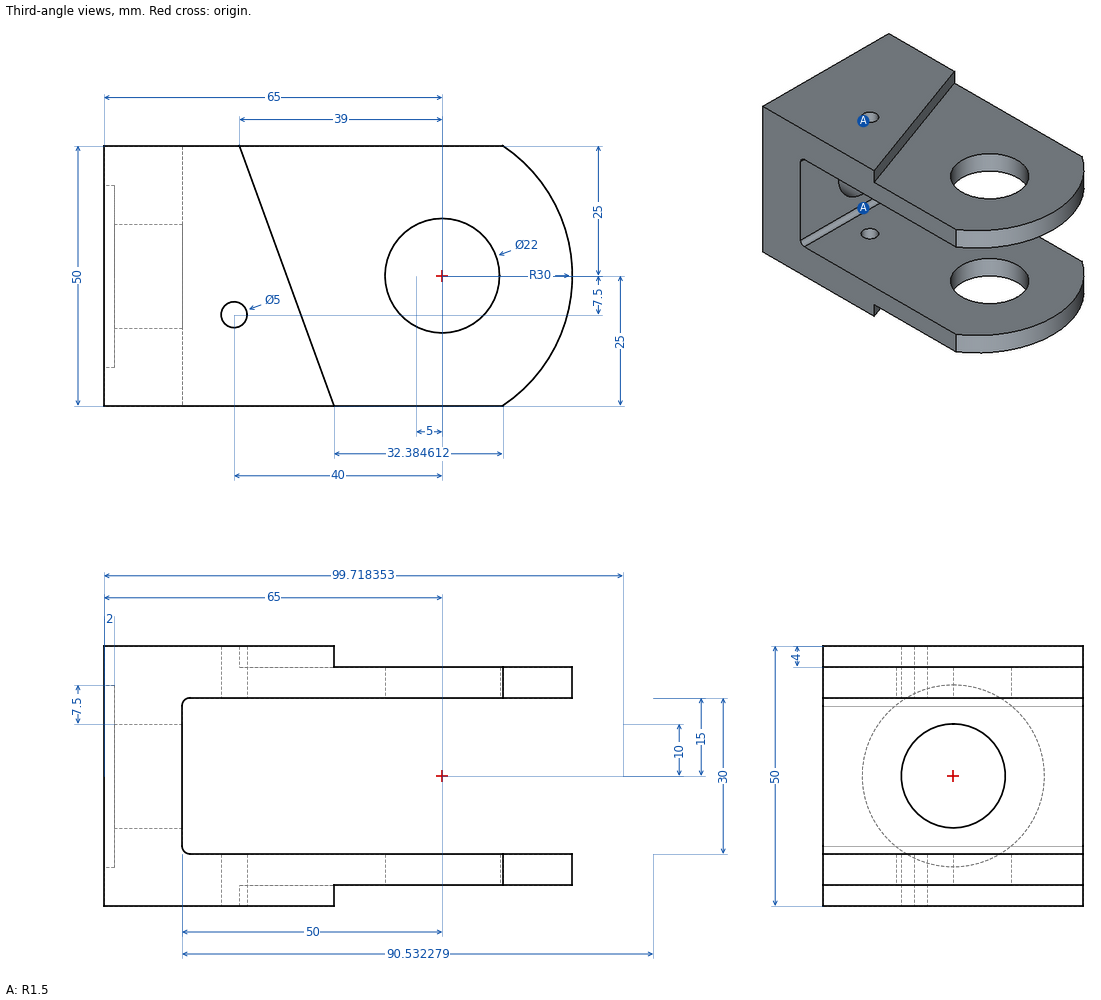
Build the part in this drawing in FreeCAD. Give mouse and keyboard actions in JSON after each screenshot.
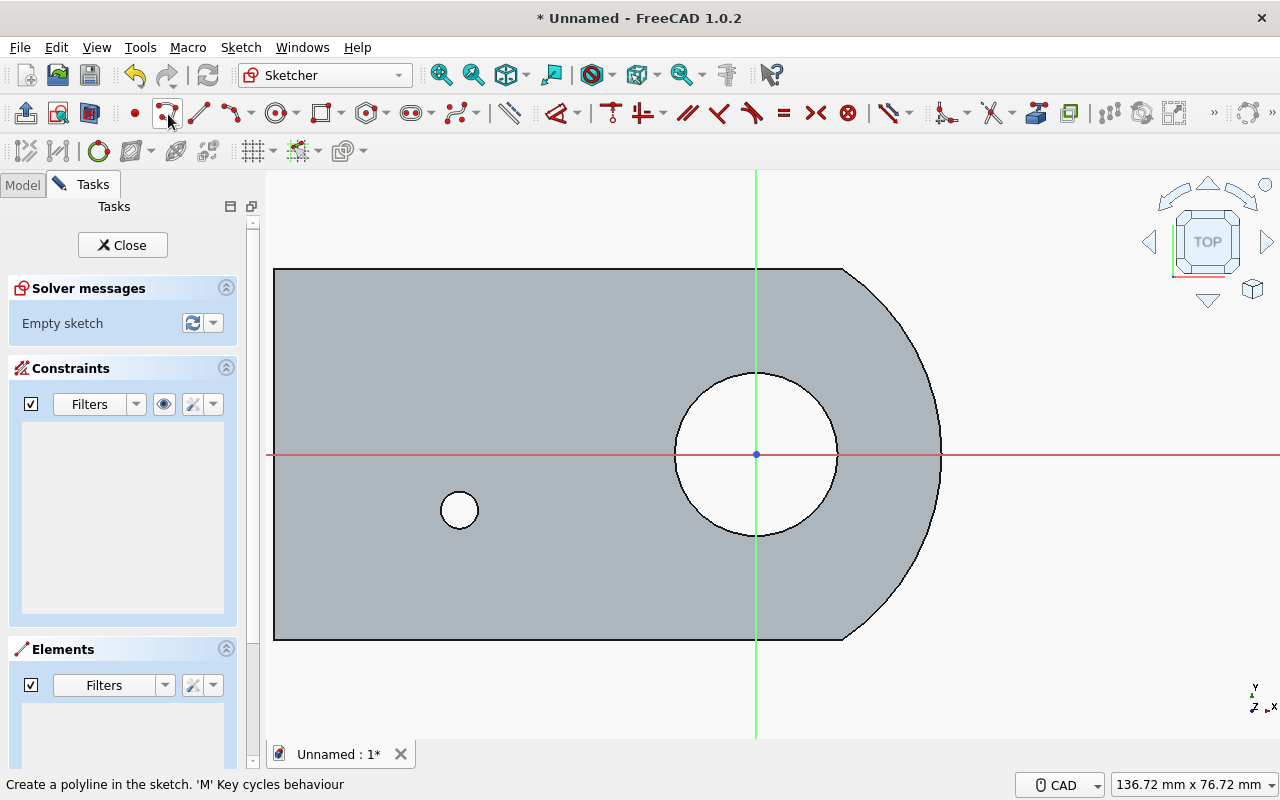
{"action": "left_click", "coordinate": [842, 269]}
{"action": "left_click", "coordinate": [467, 269]}
{"action": "left_click", "coordinate": [602, 640]}
{"action": "left_click", "coordinate": [842, 640]}
{"action": "right_click", "coordinate": [842, 640]}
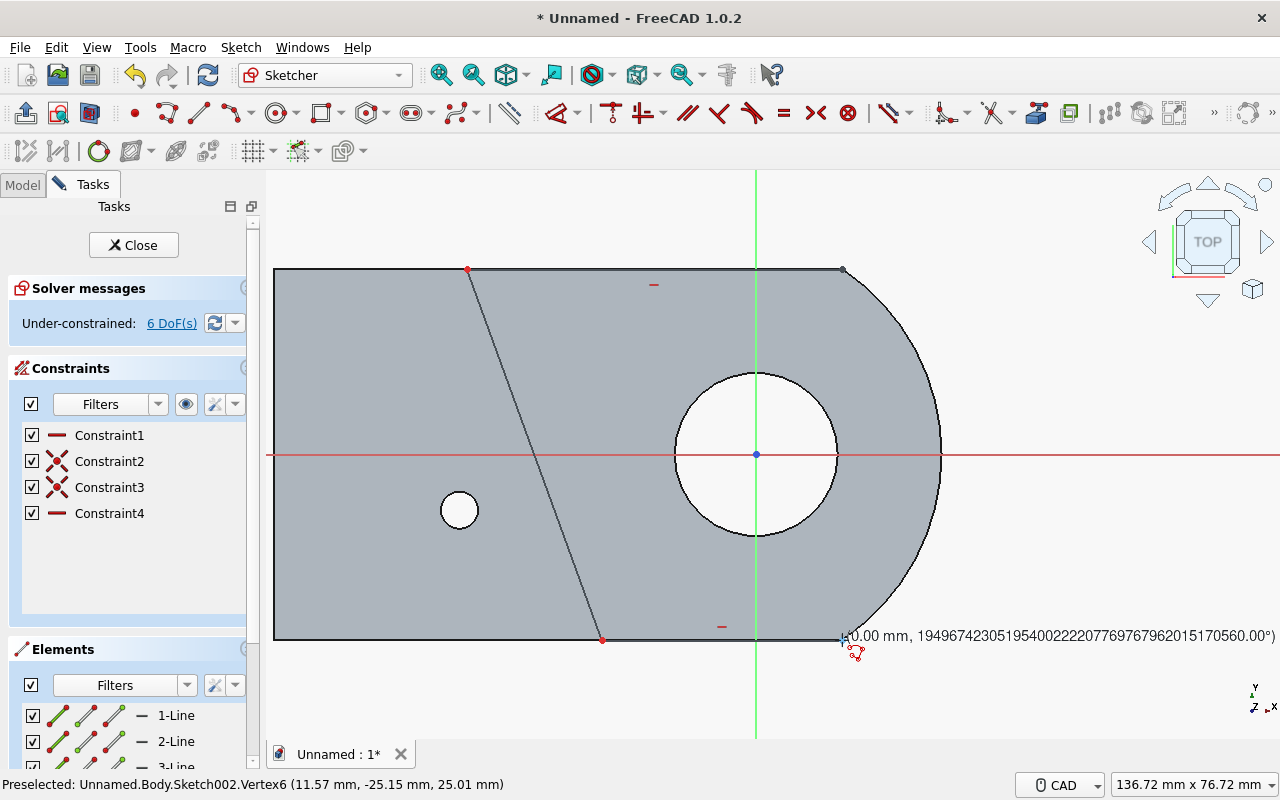
{"action": "left_click", "coordinate": [232, 114]}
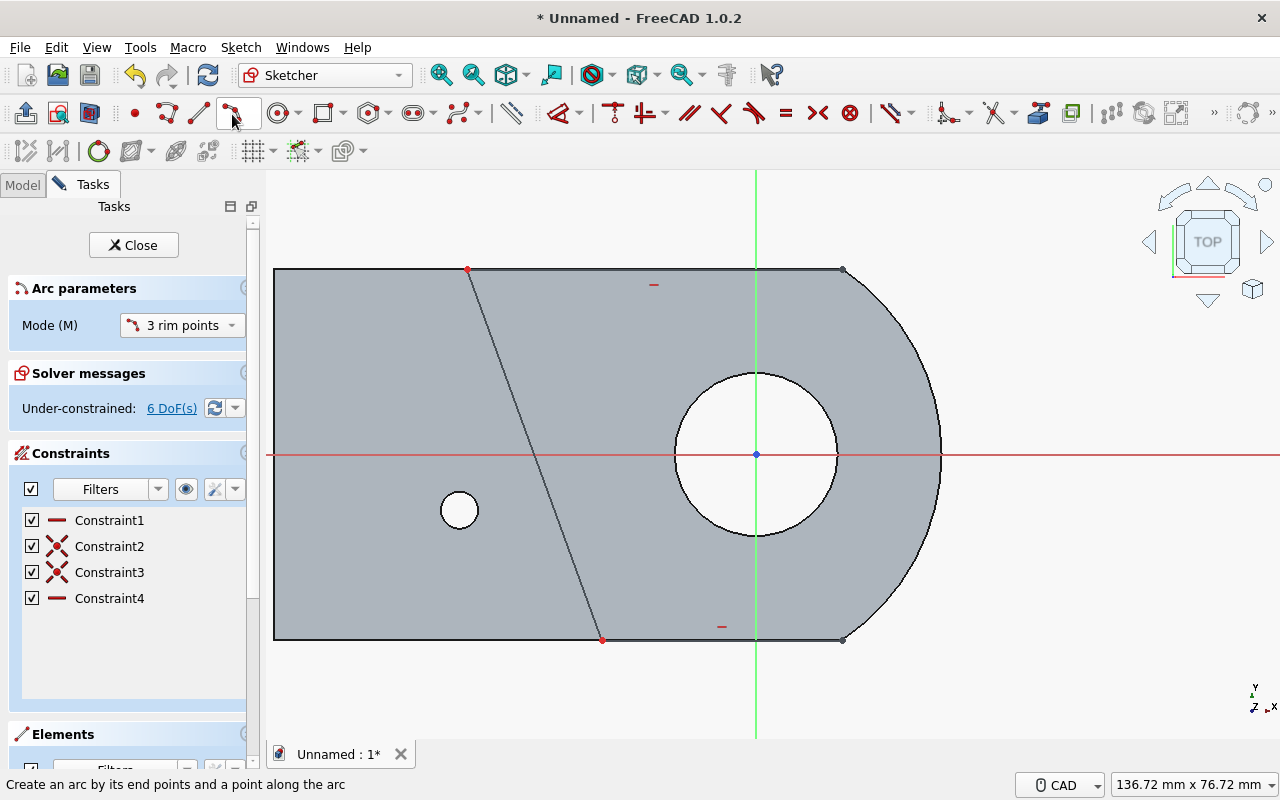
{"action": "left_click", "coordinate": [842, 641]}
{"action": "left_click", "coordinate": [842, 270]}
{"action": "left_click", "coordinate": [937, 498]}
{"action": "key", "text": "Escape"}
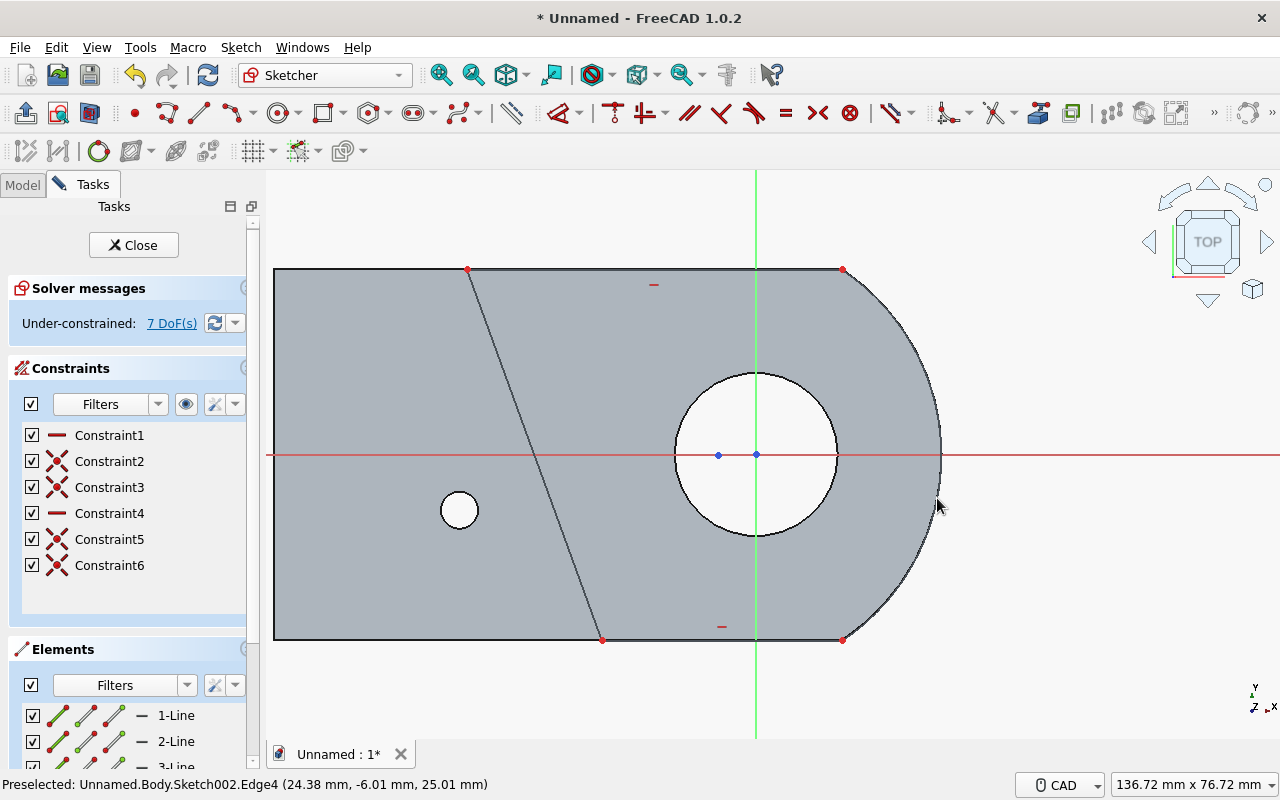
{"action": "left_click", "coordinate": [718, 455]}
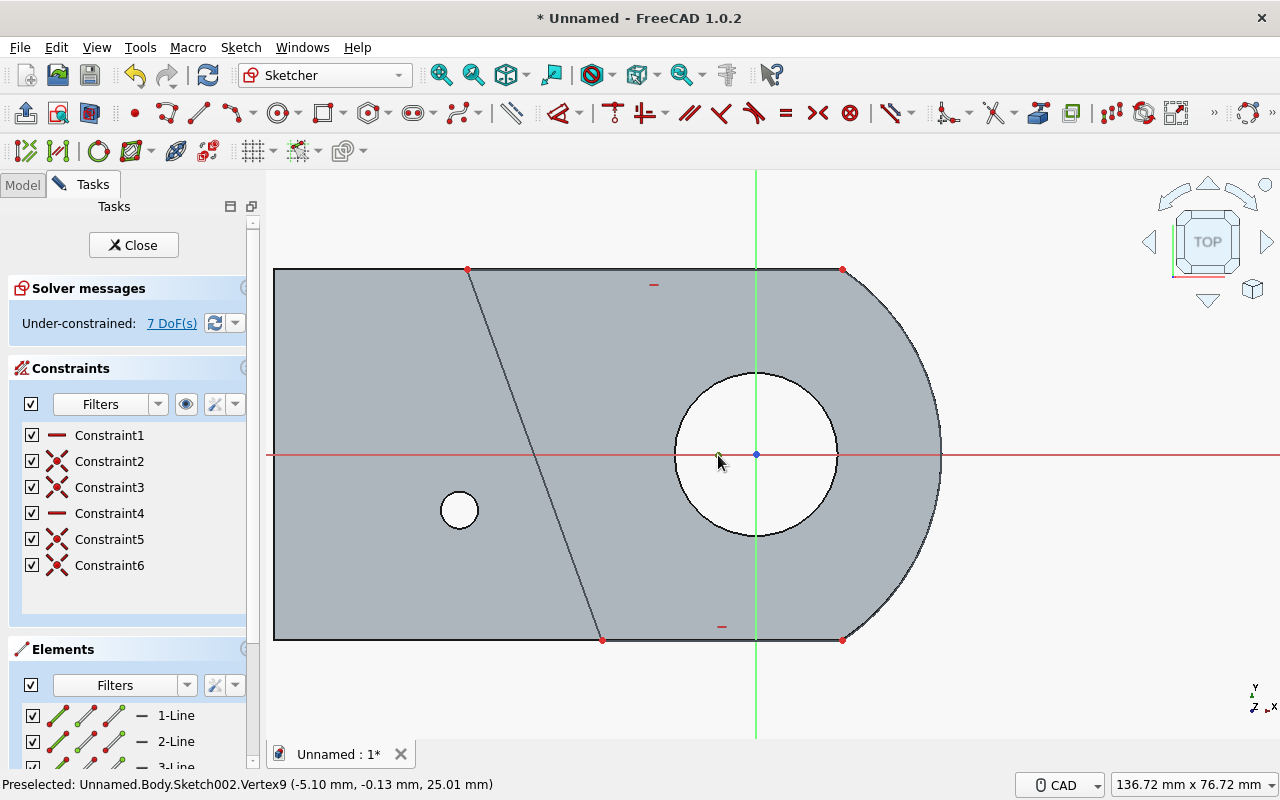
{"action": "left_click", "coordinate": [353, 454]}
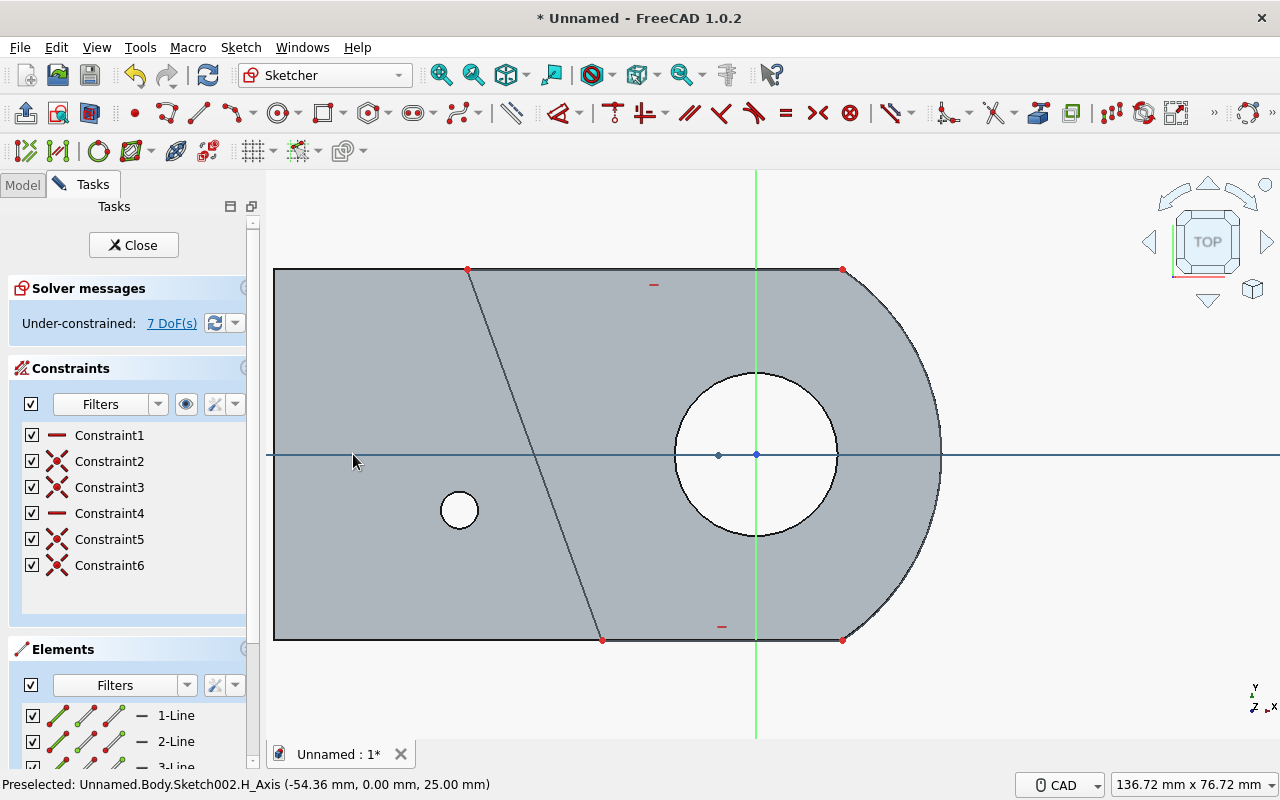
{"action": "left_click", "coordinate": [614, 114]}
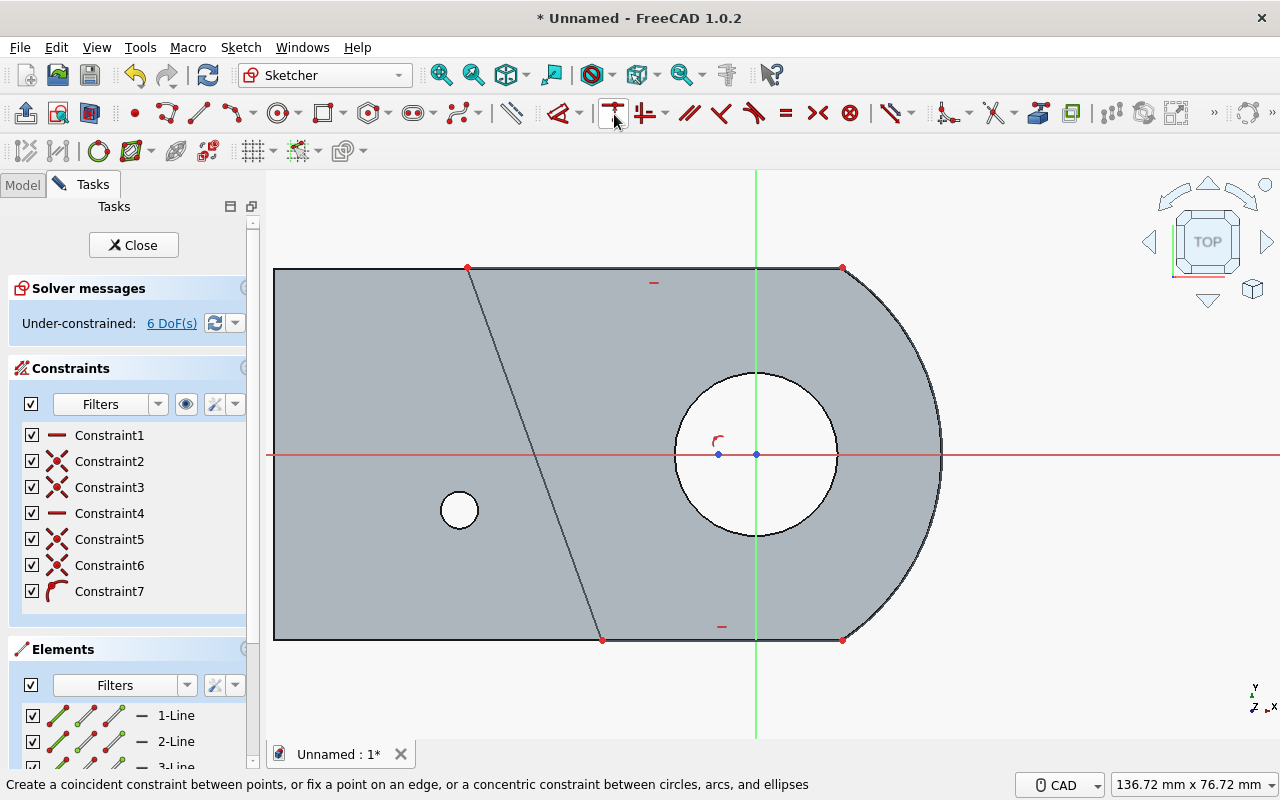
{"action": "left_click", "coordinate": [558, 114]}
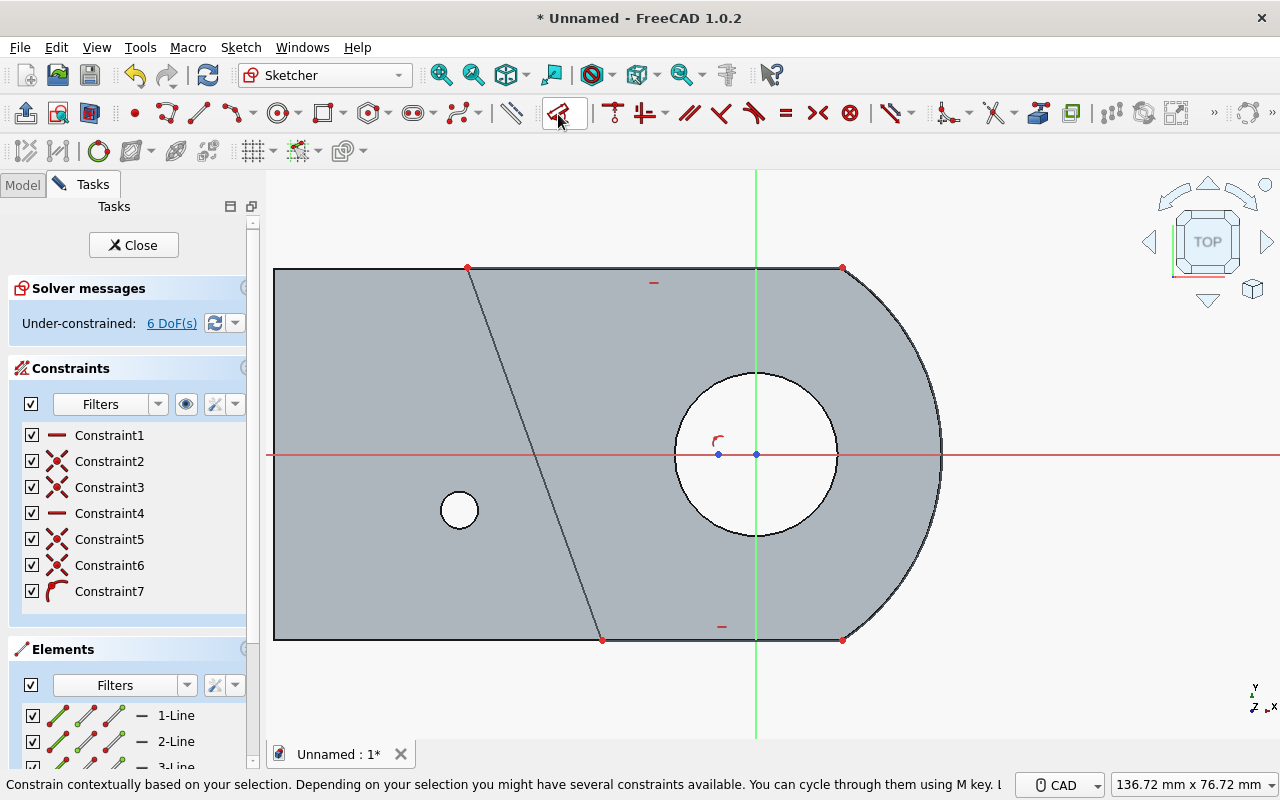
{"action": "left_click", "coordinate": [925, 540]}
{"action": "left_click", "coordinate": [955, 552]}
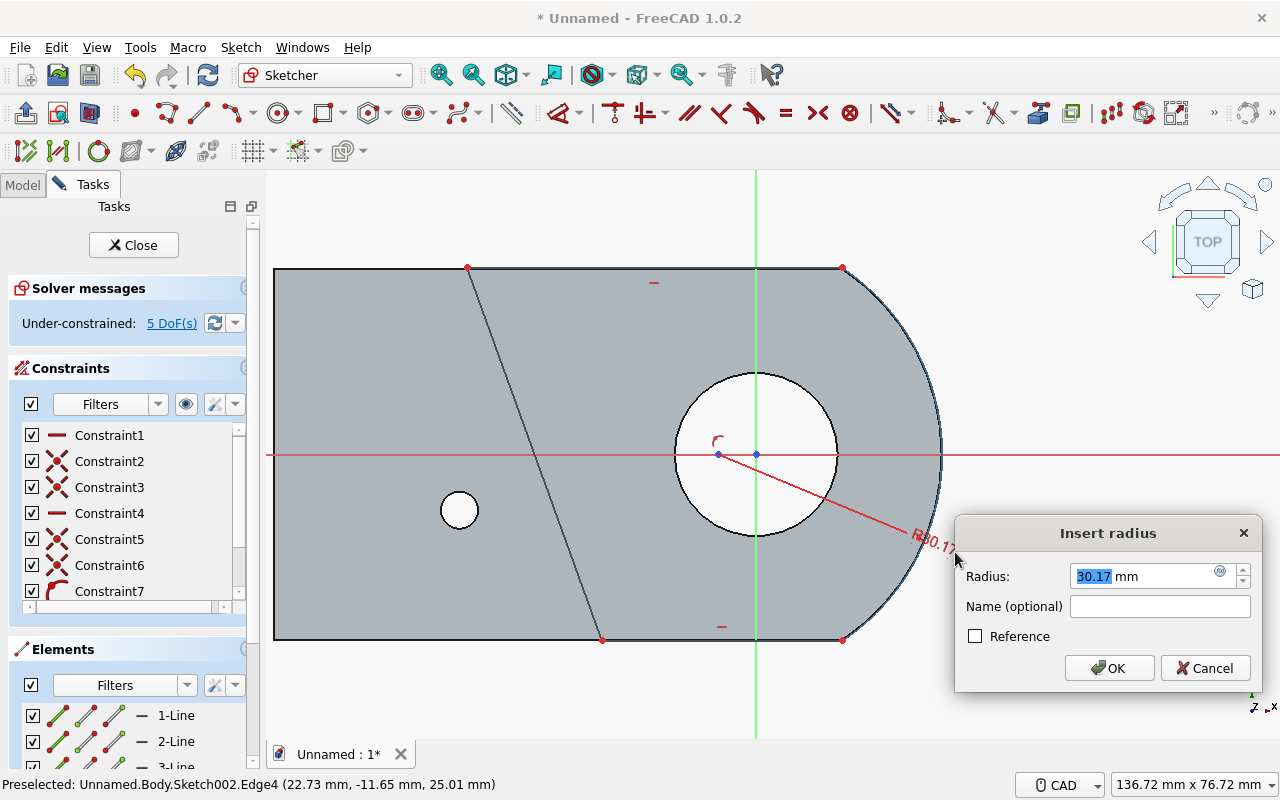
{"action": "type", "text": "30"}
{"action": "key", "text": "Return"}